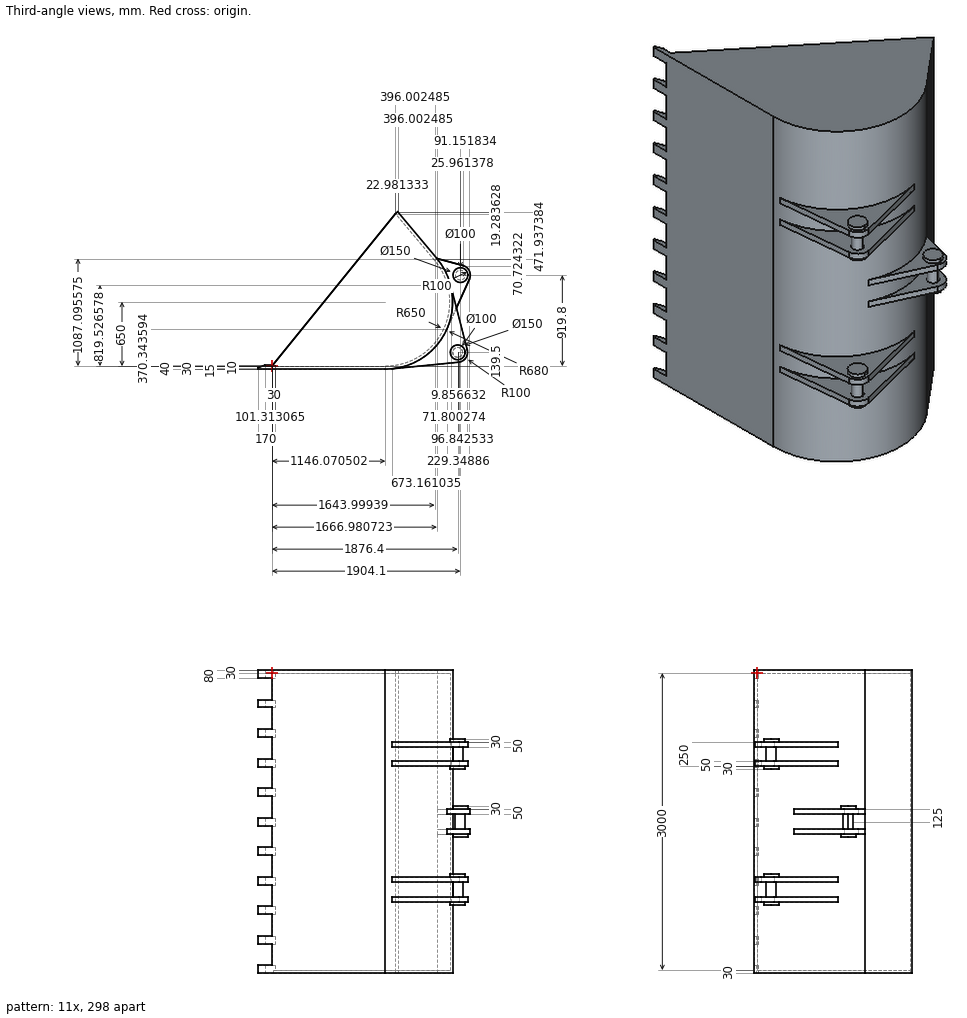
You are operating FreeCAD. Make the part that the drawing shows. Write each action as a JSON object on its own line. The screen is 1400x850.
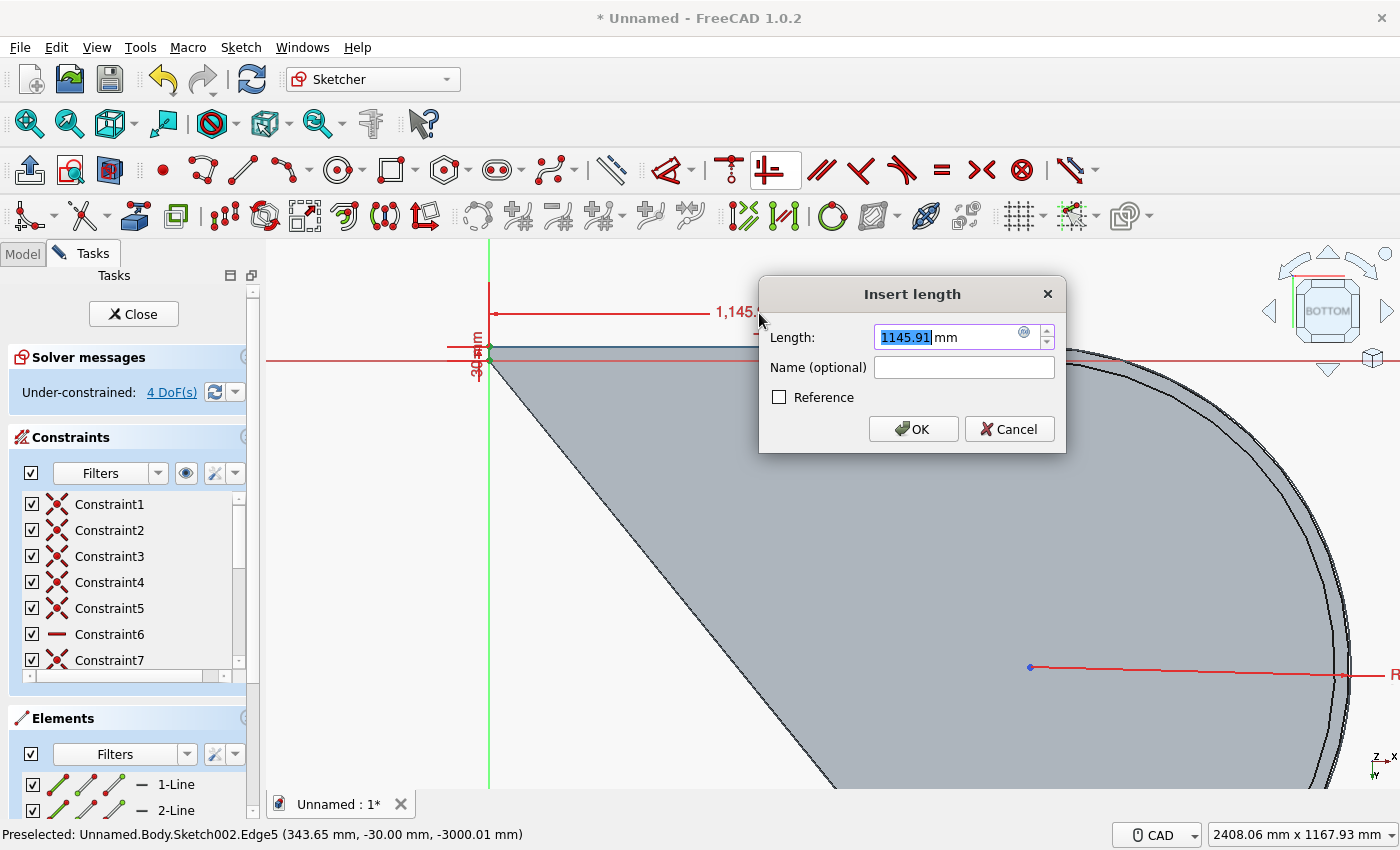
{"action": "type", "text": "1146.070502"}
{"action": "key", "text": "Return"}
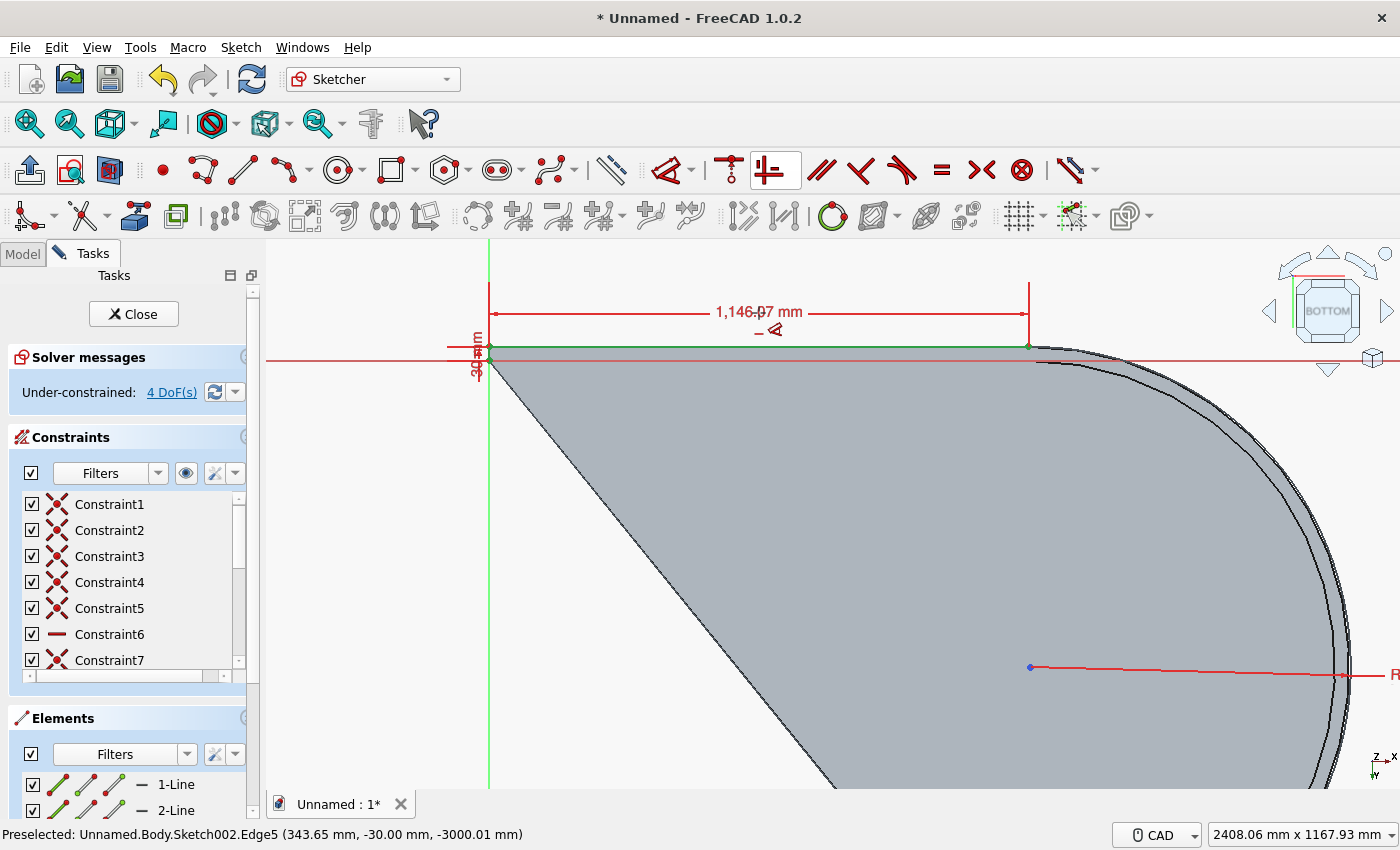
{"action": "scroll", "coordinate": [651, 345], "scroll_direction": "down", "scroll_amount": 4}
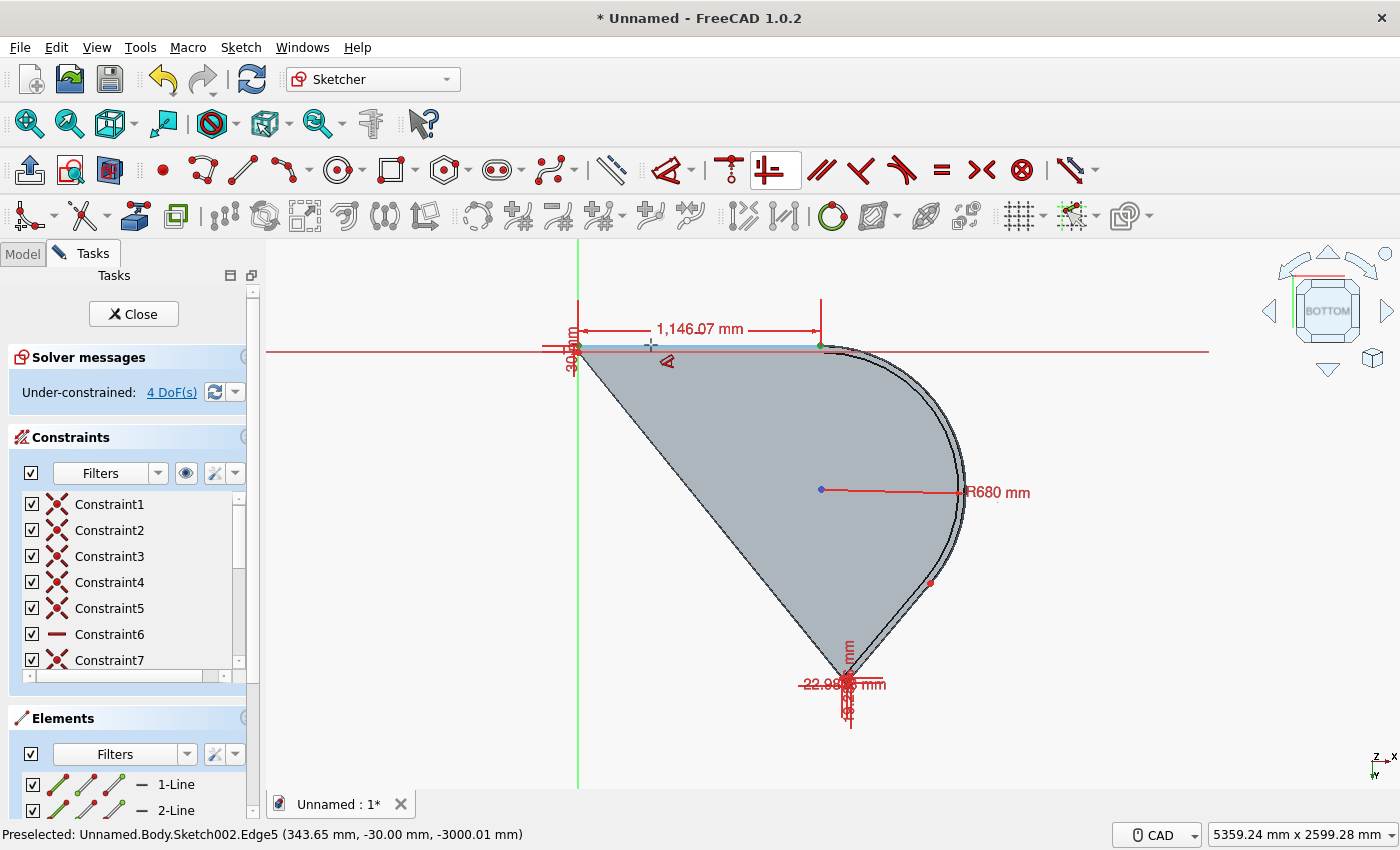
{"action": "left_click", "coordinate": [906, 613]}
{"action": "left_click", "coordinate": [889, 717]}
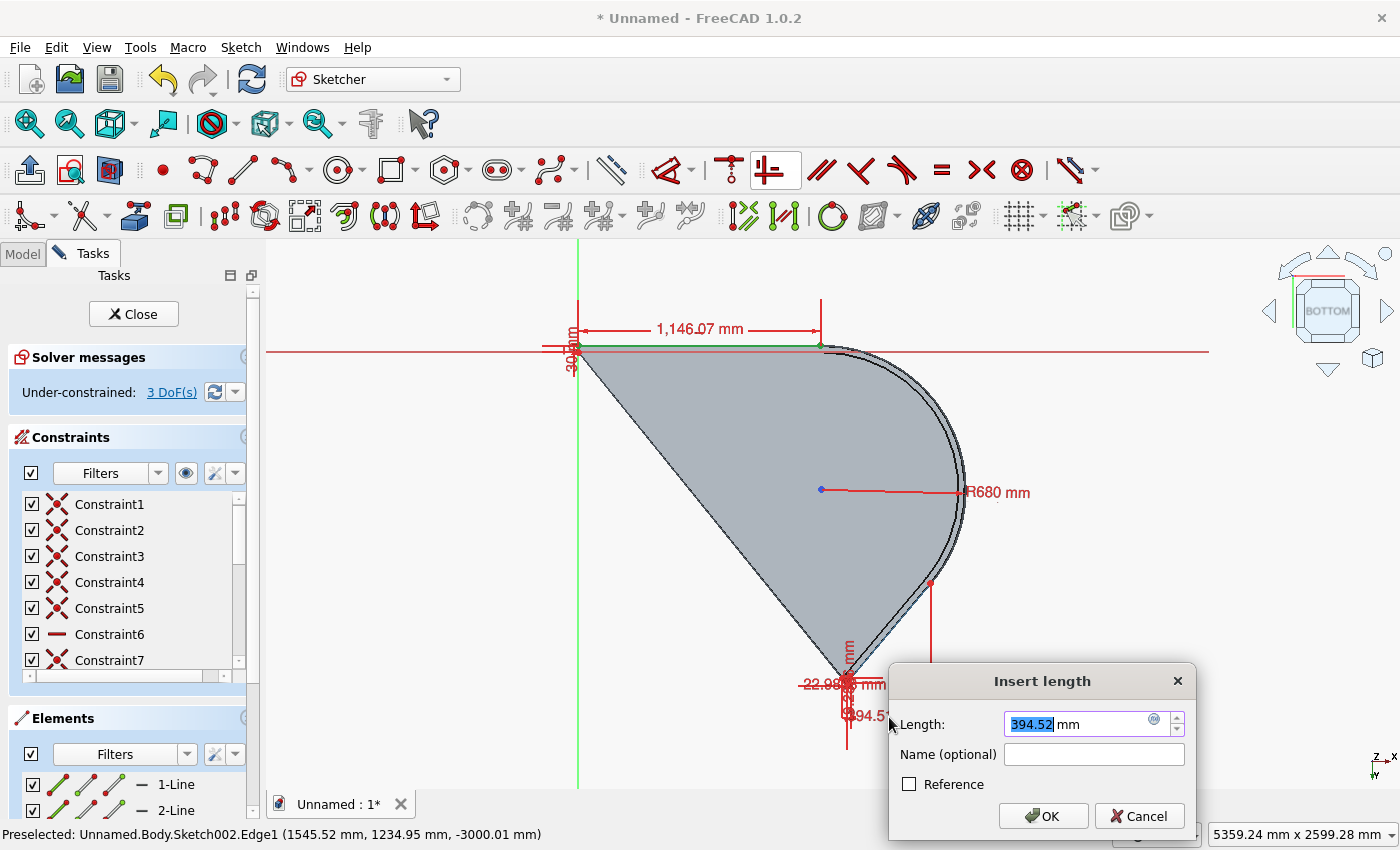
{"action": "type", "text": "396.002485"}
{"action": "key", "text": "Return"}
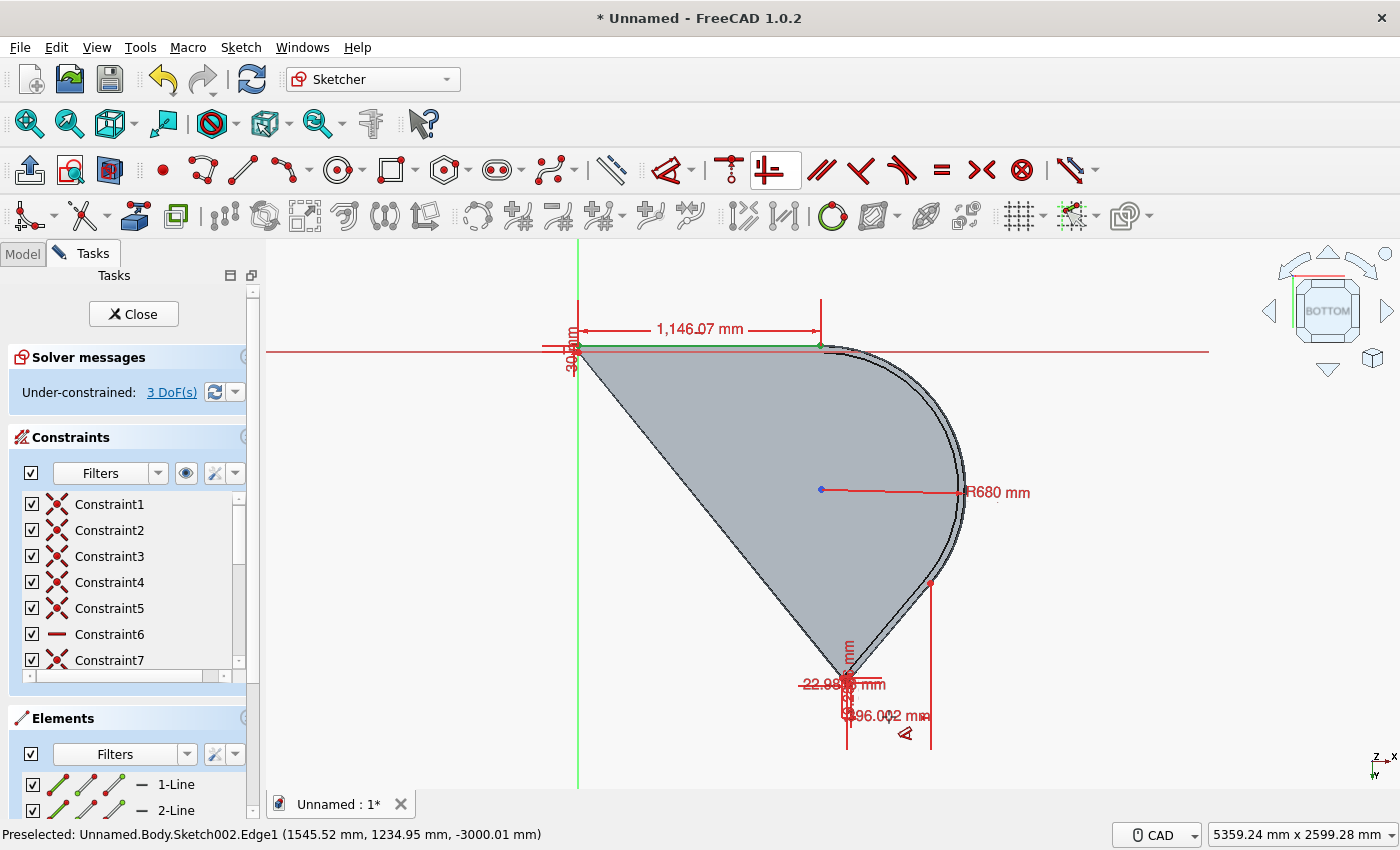
{"action": "left_click", "coordinate": [906, 613]}
{"action": "left_click", "coordinate": [965, 633]}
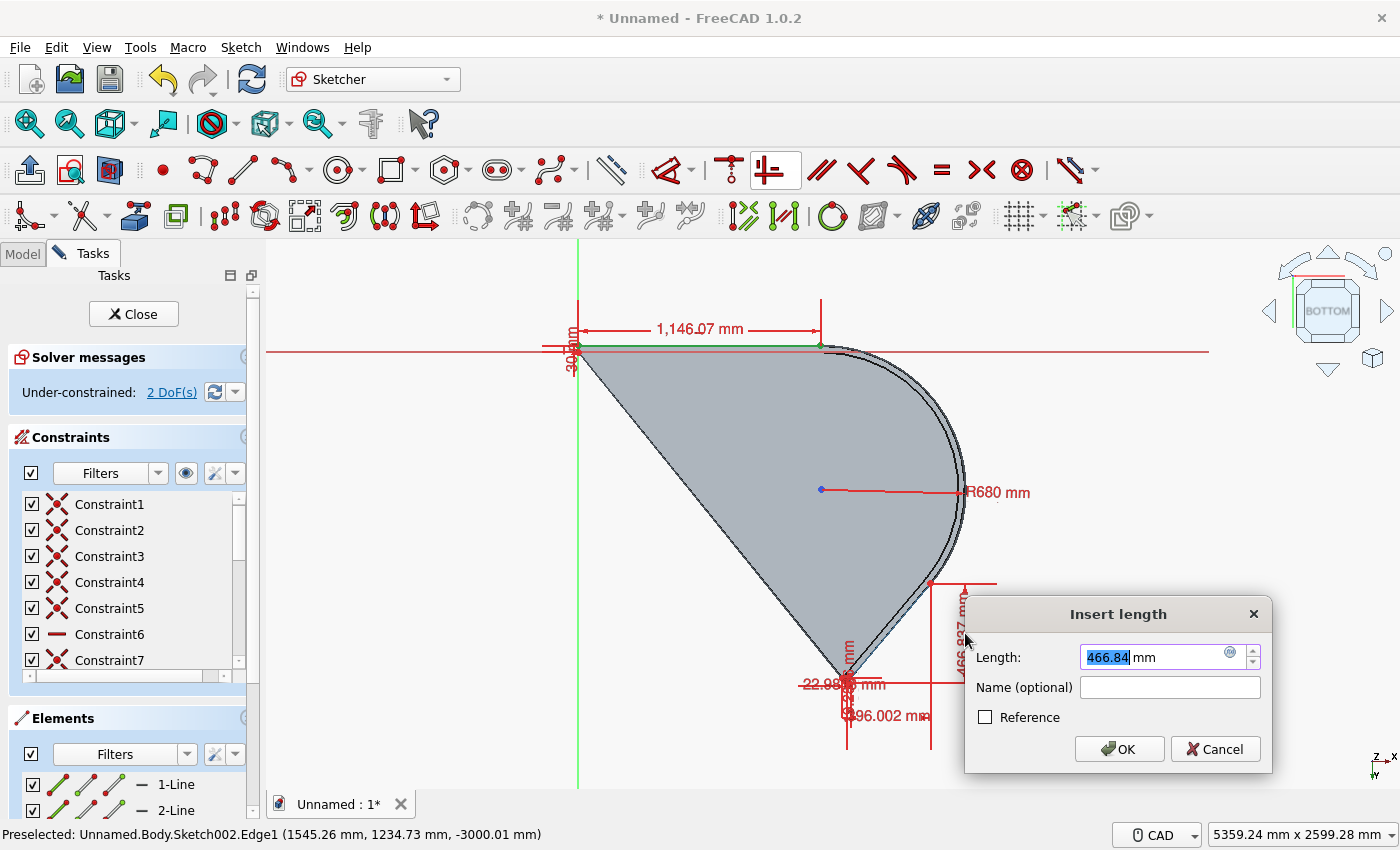
{"action": "type", "text": "471.937384"}
{"action": "key", "text": "Return"}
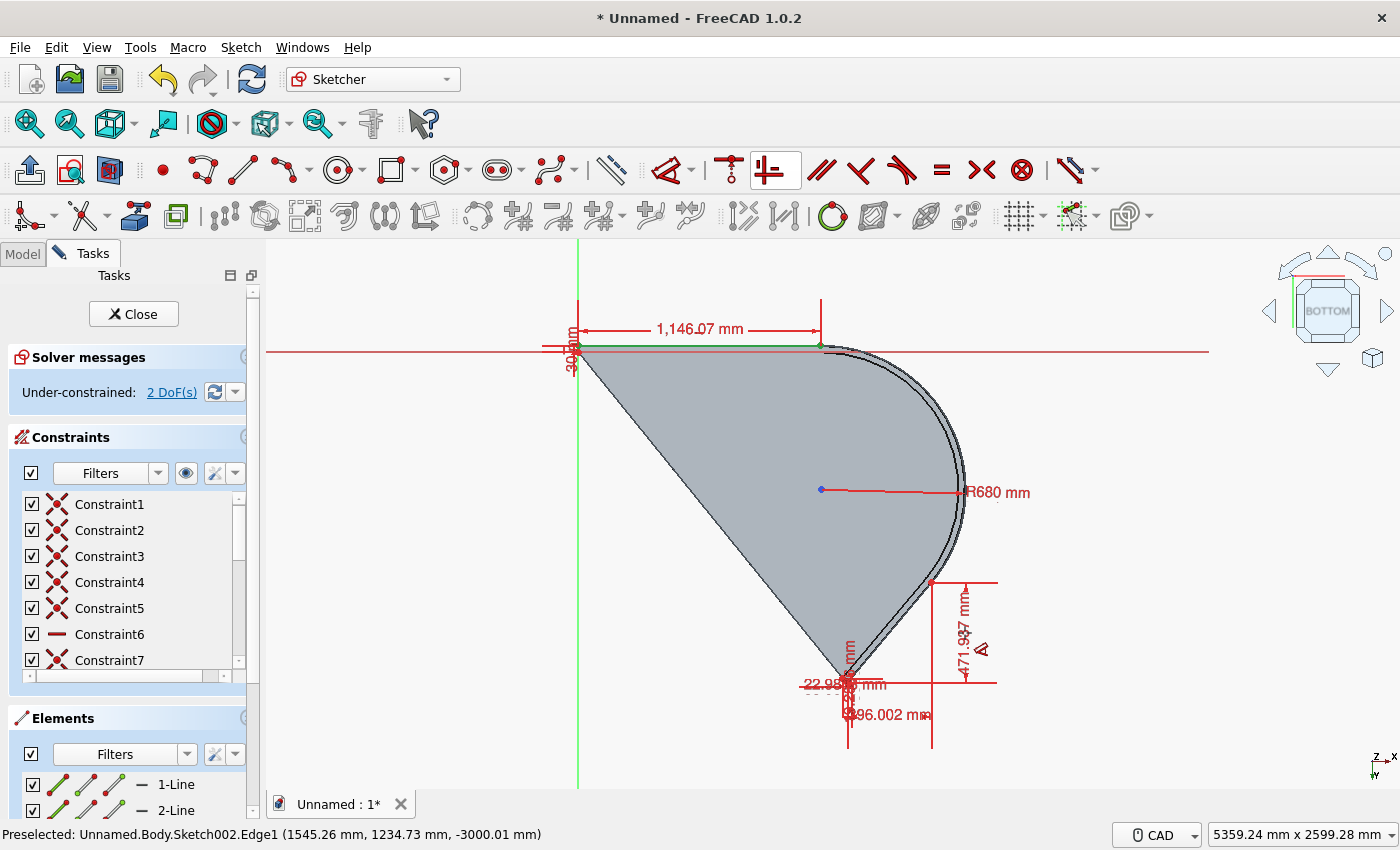
{"action": "left_click", "coordinate": [932, 583]}
{"action": "left_click", "coordinate": [836, 318]}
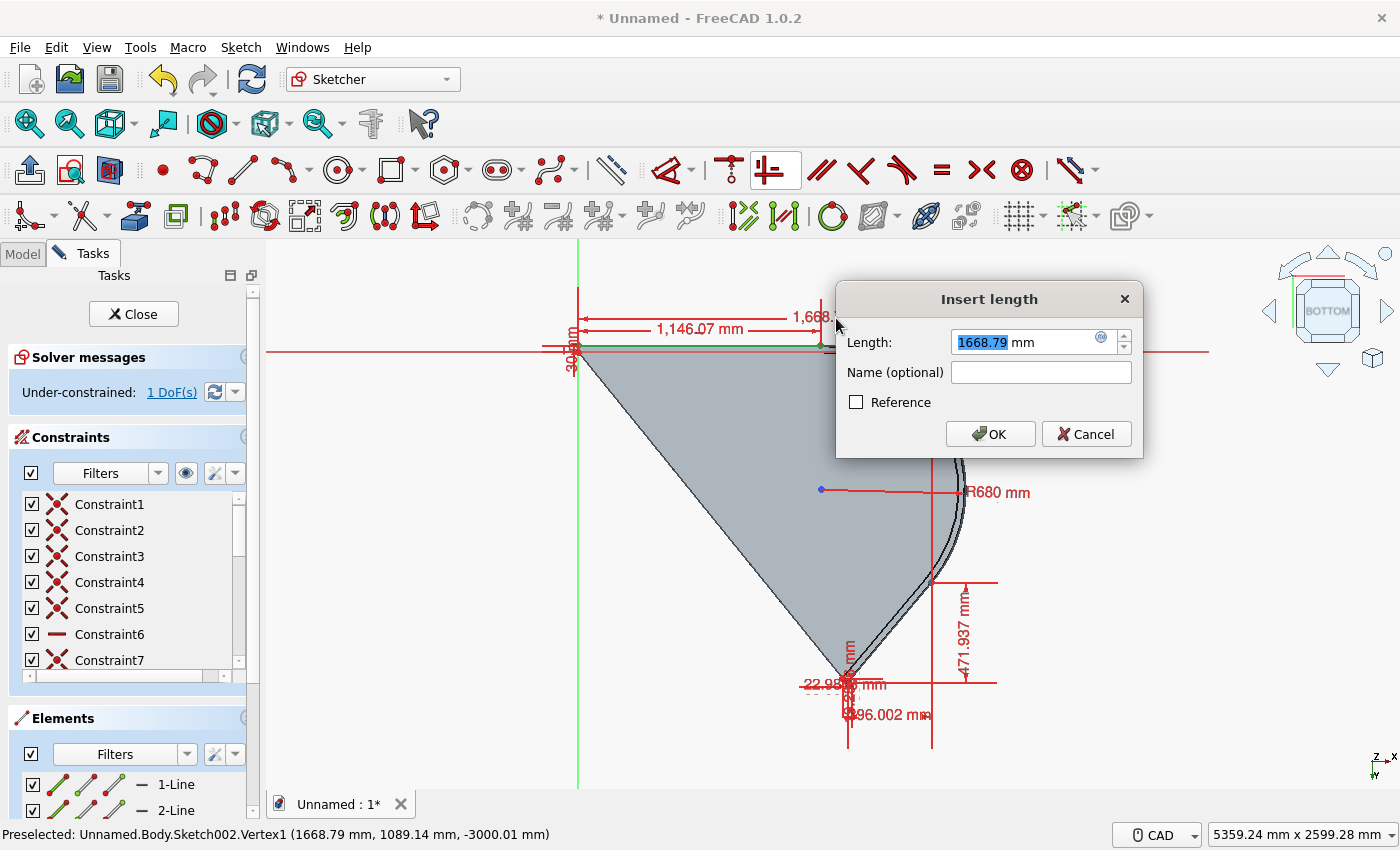
{"action": "type", "text": "1666.980723"}
{"action": "key", "text": "Return"}